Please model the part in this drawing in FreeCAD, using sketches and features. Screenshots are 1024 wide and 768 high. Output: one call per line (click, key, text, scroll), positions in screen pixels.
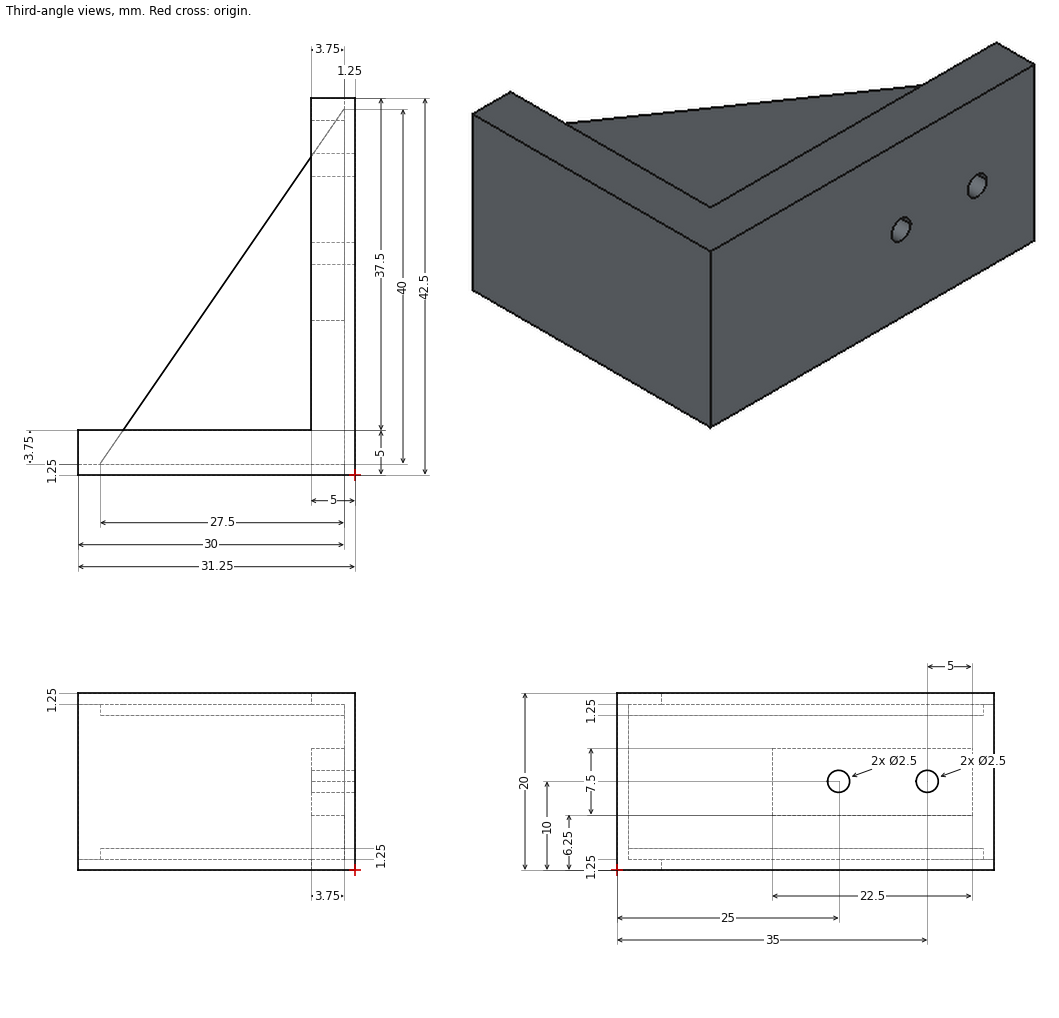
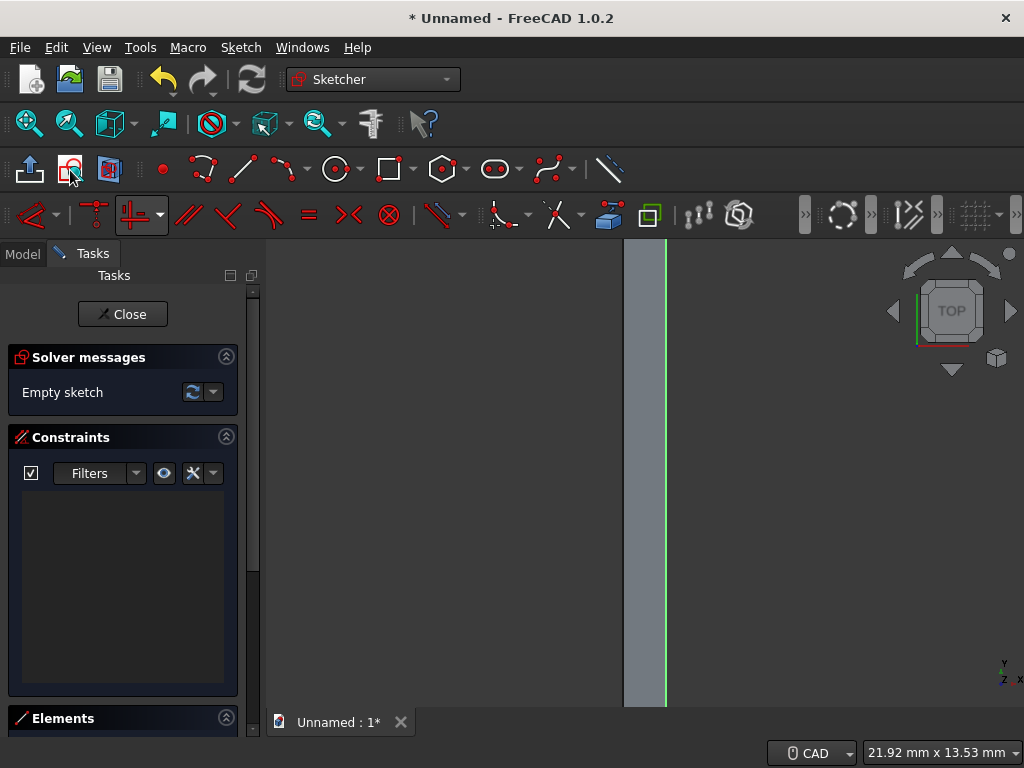
scroll(691, 542, down, 8)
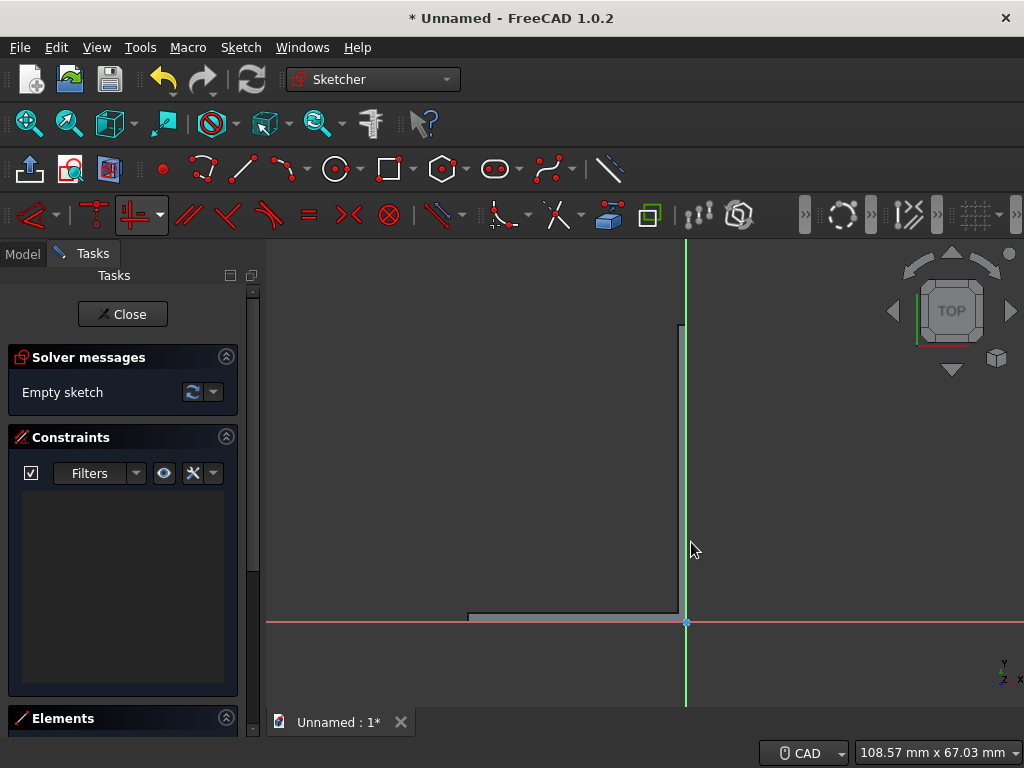
click(204, 170)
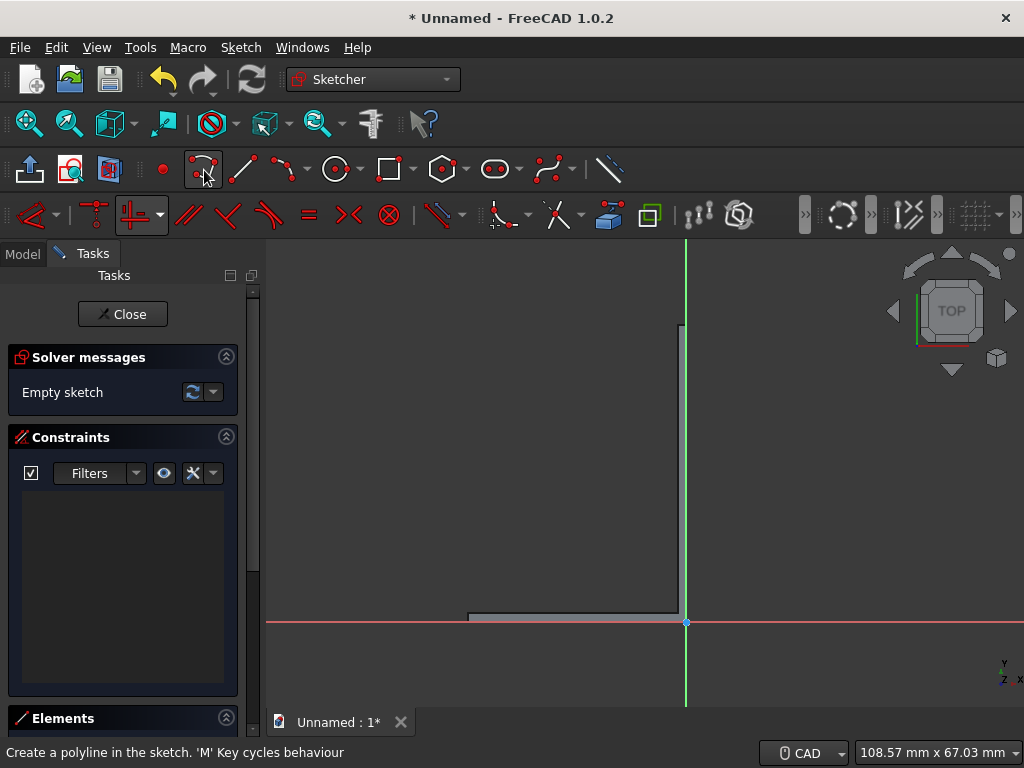
scroll(678, 613, up, 3)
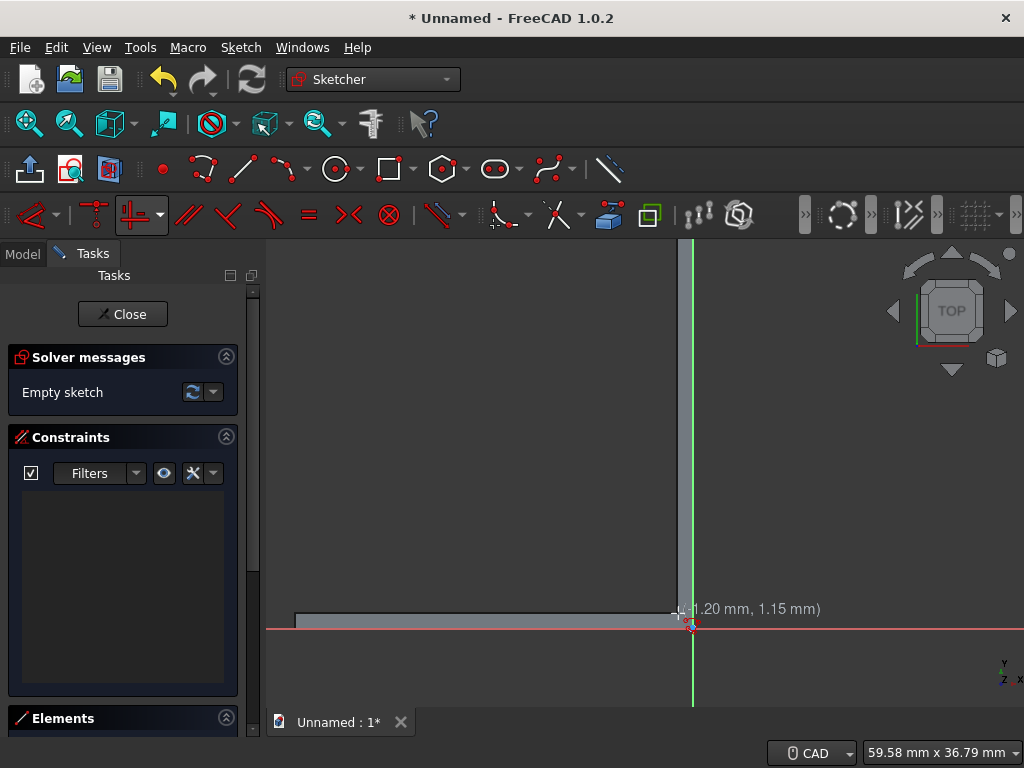
click(677, 613)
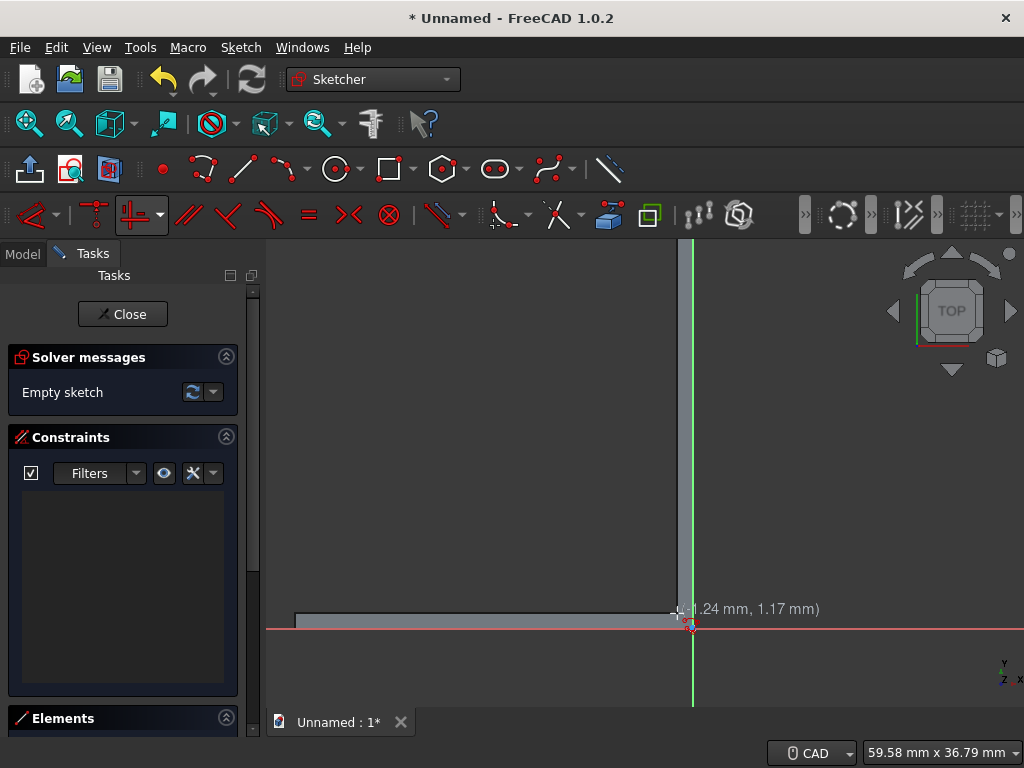
scroll(677, 612, down, 3)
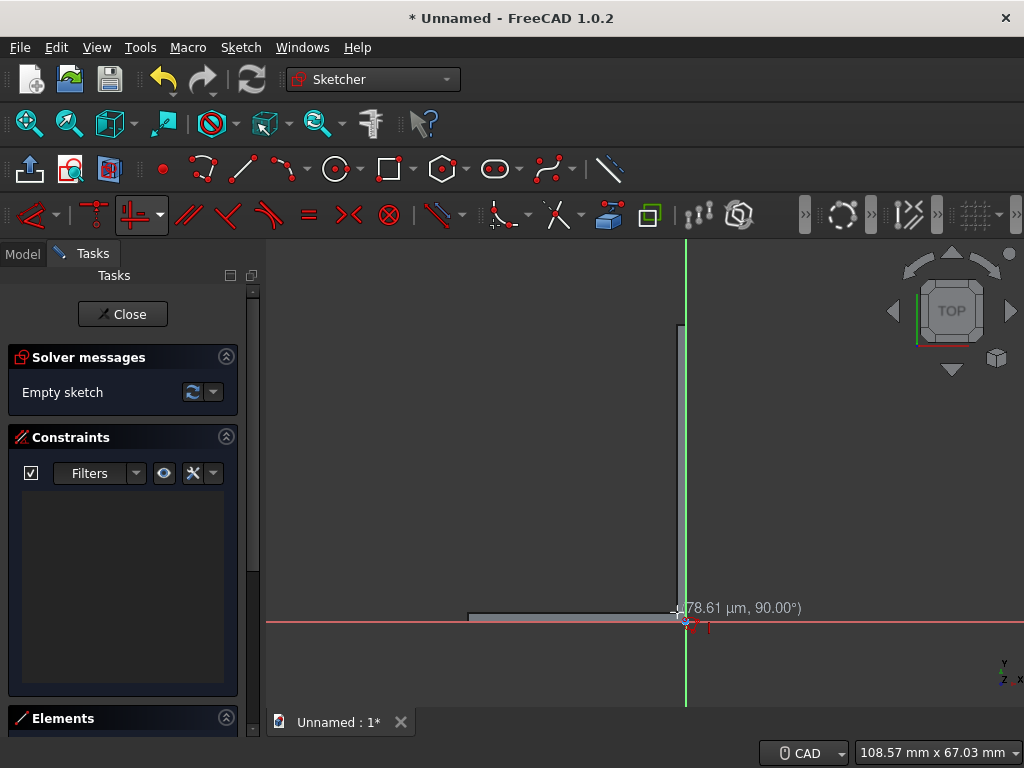
scroll(677, 325, up, 3)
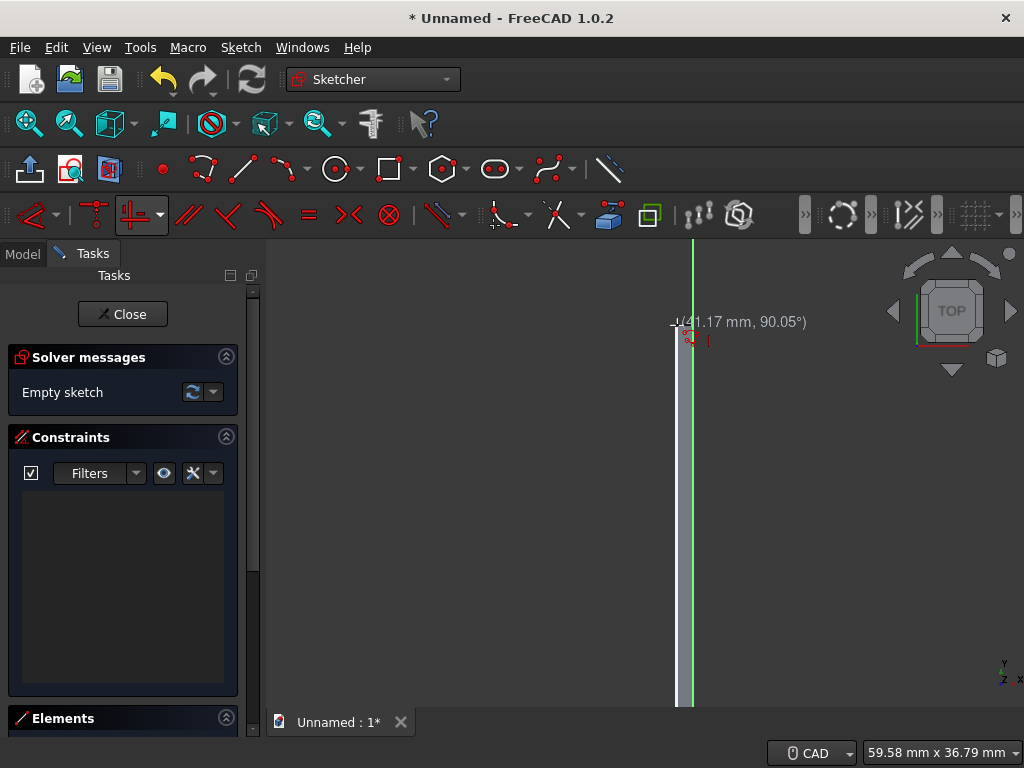
click(677, 325)
click(629, 325)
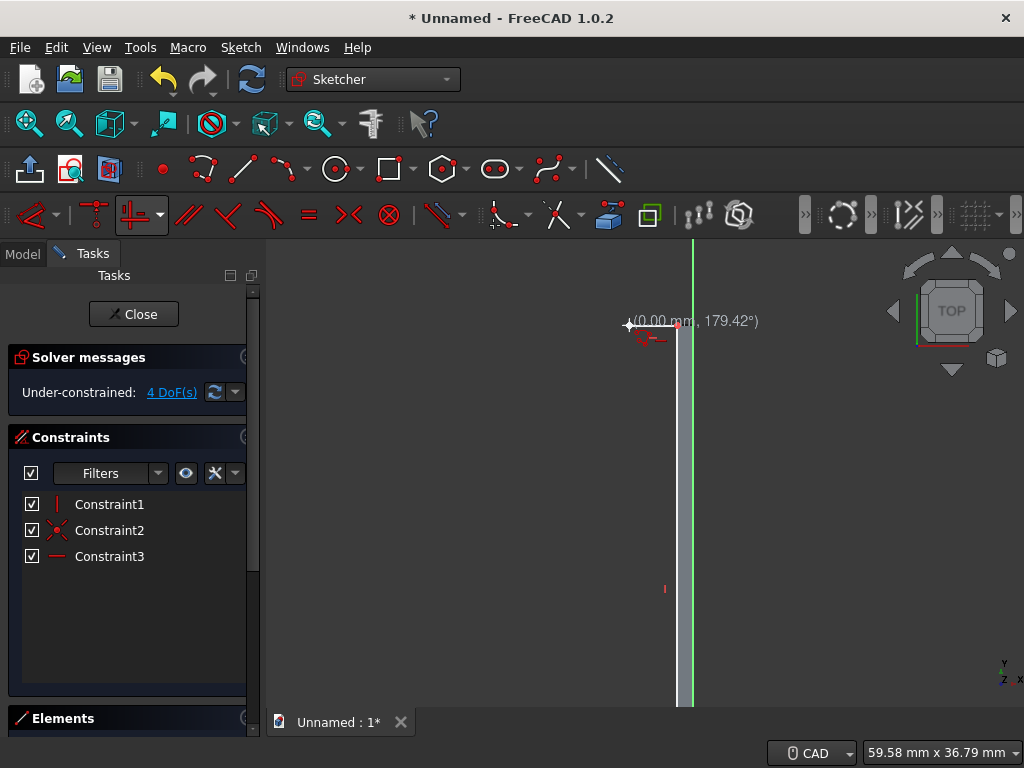
scroll(677, 325, down, 3)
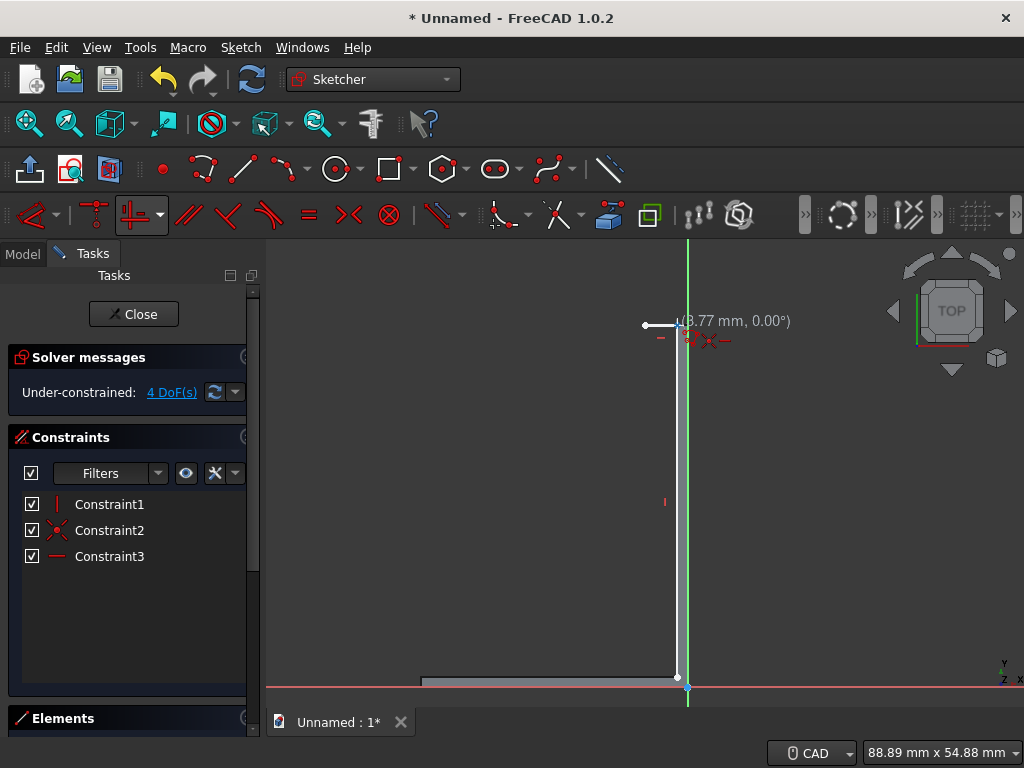
click(651, 587)
click(468, 587)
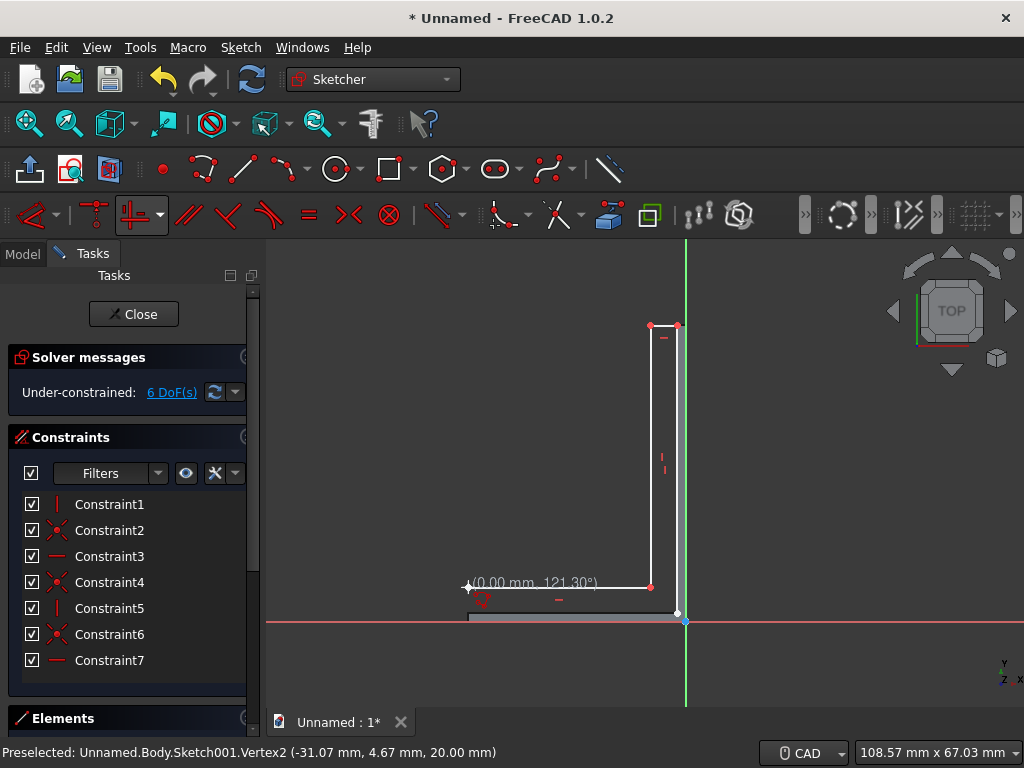
scroll(468, 613, up, 3)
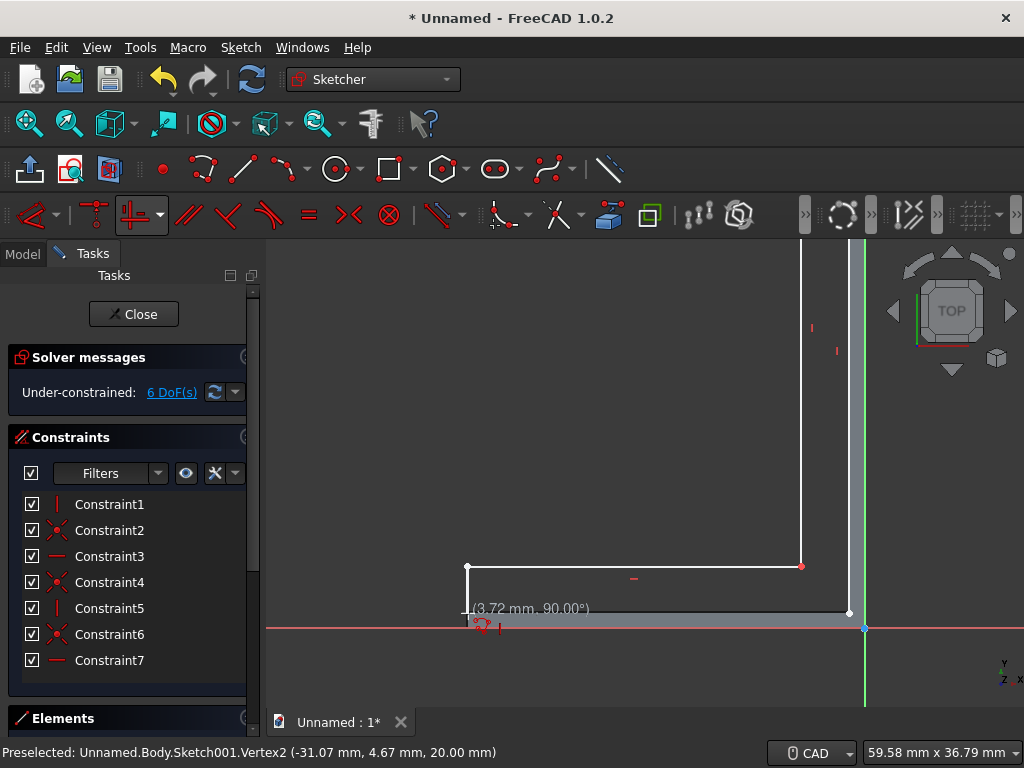
click(468, 612)
click(849, 613)
key(Escape)
key(Escape)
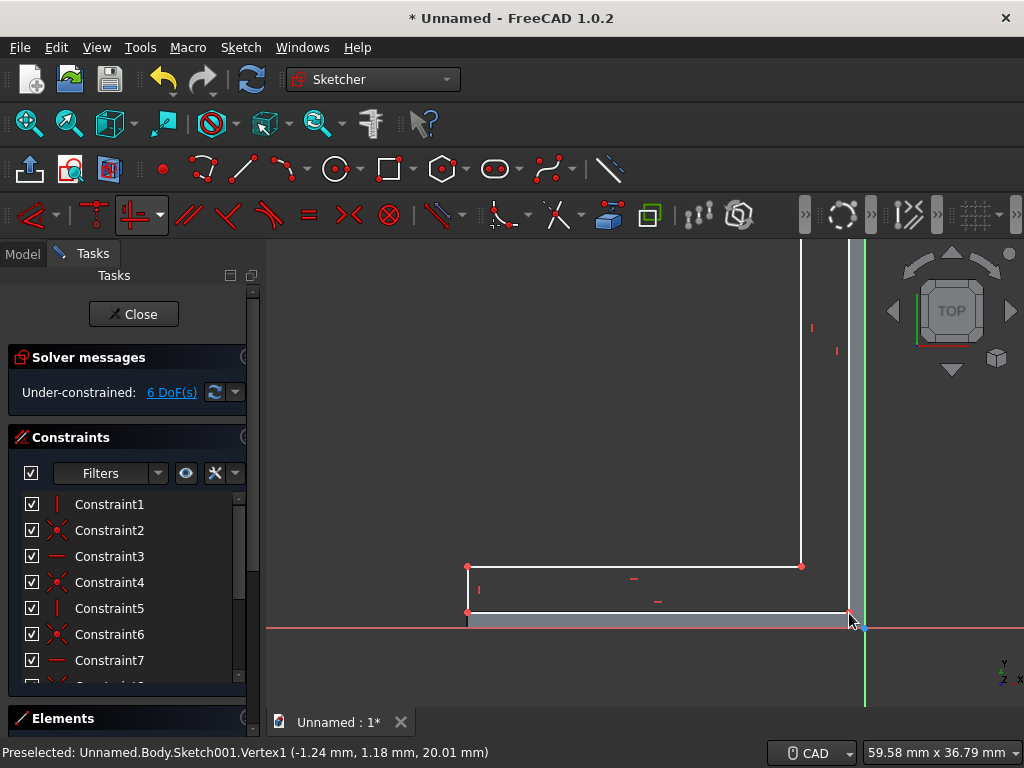
click(32, 216)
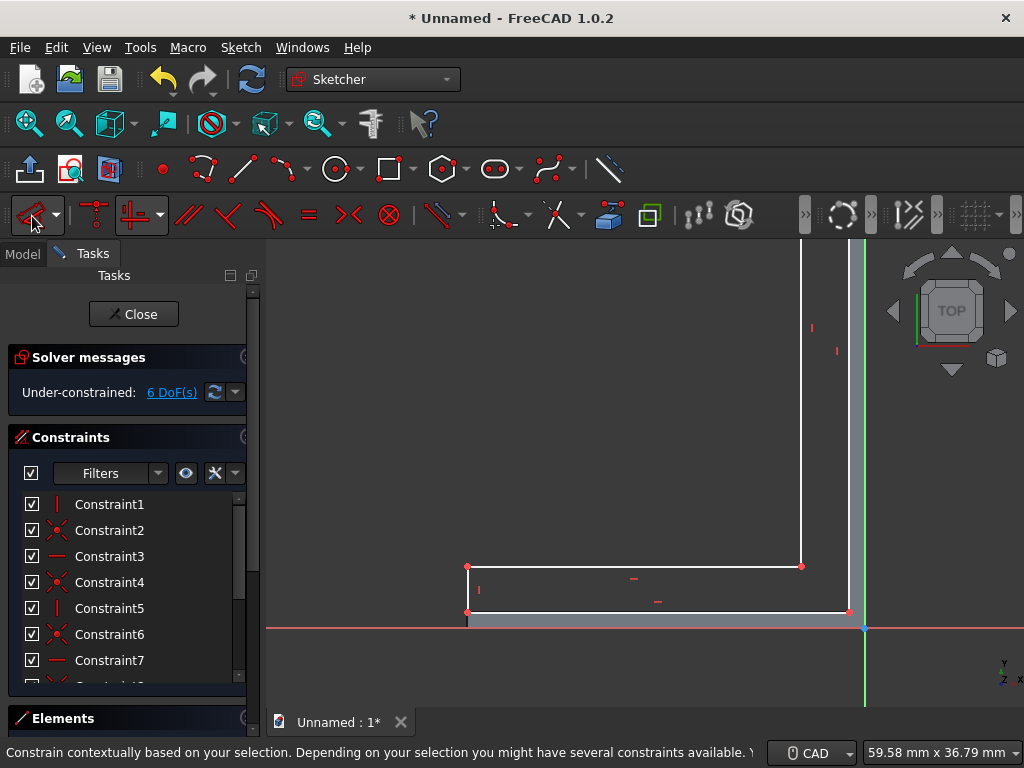
click(582, 613)
click(658, 647)